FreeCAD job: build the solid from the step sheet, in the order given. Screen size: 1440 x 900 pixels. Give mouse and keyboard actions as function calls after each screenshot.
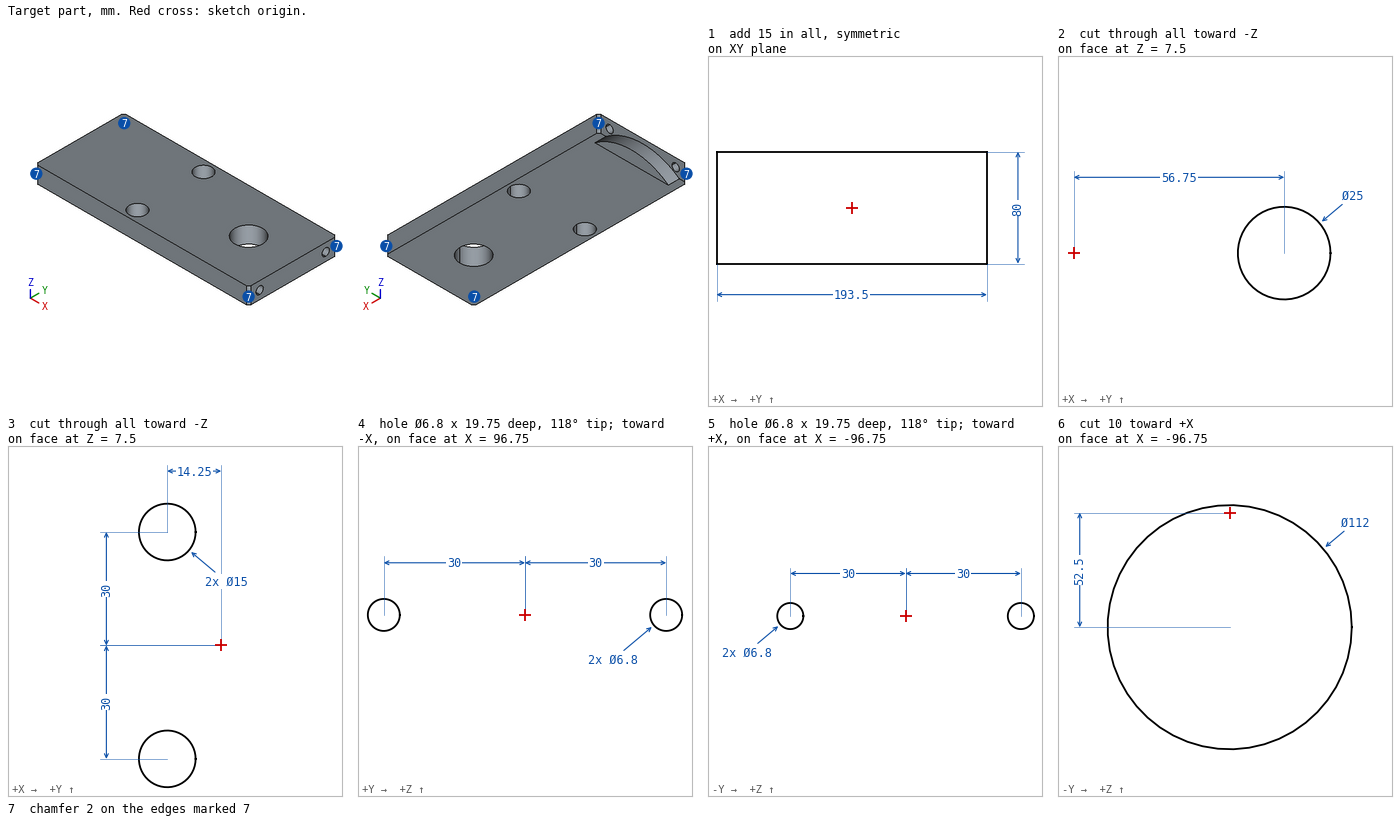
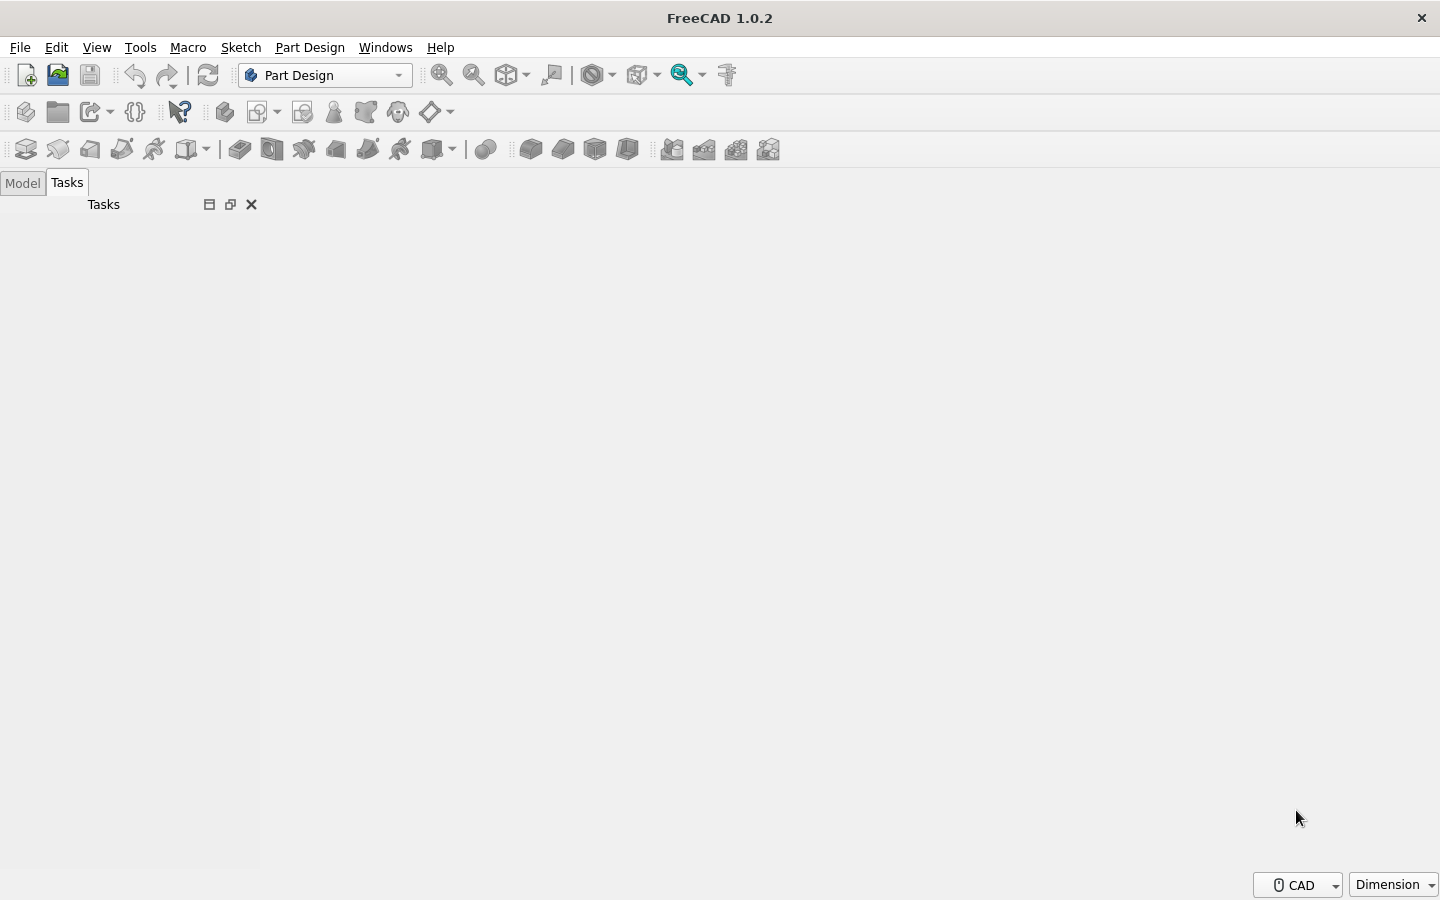
click(26, 76)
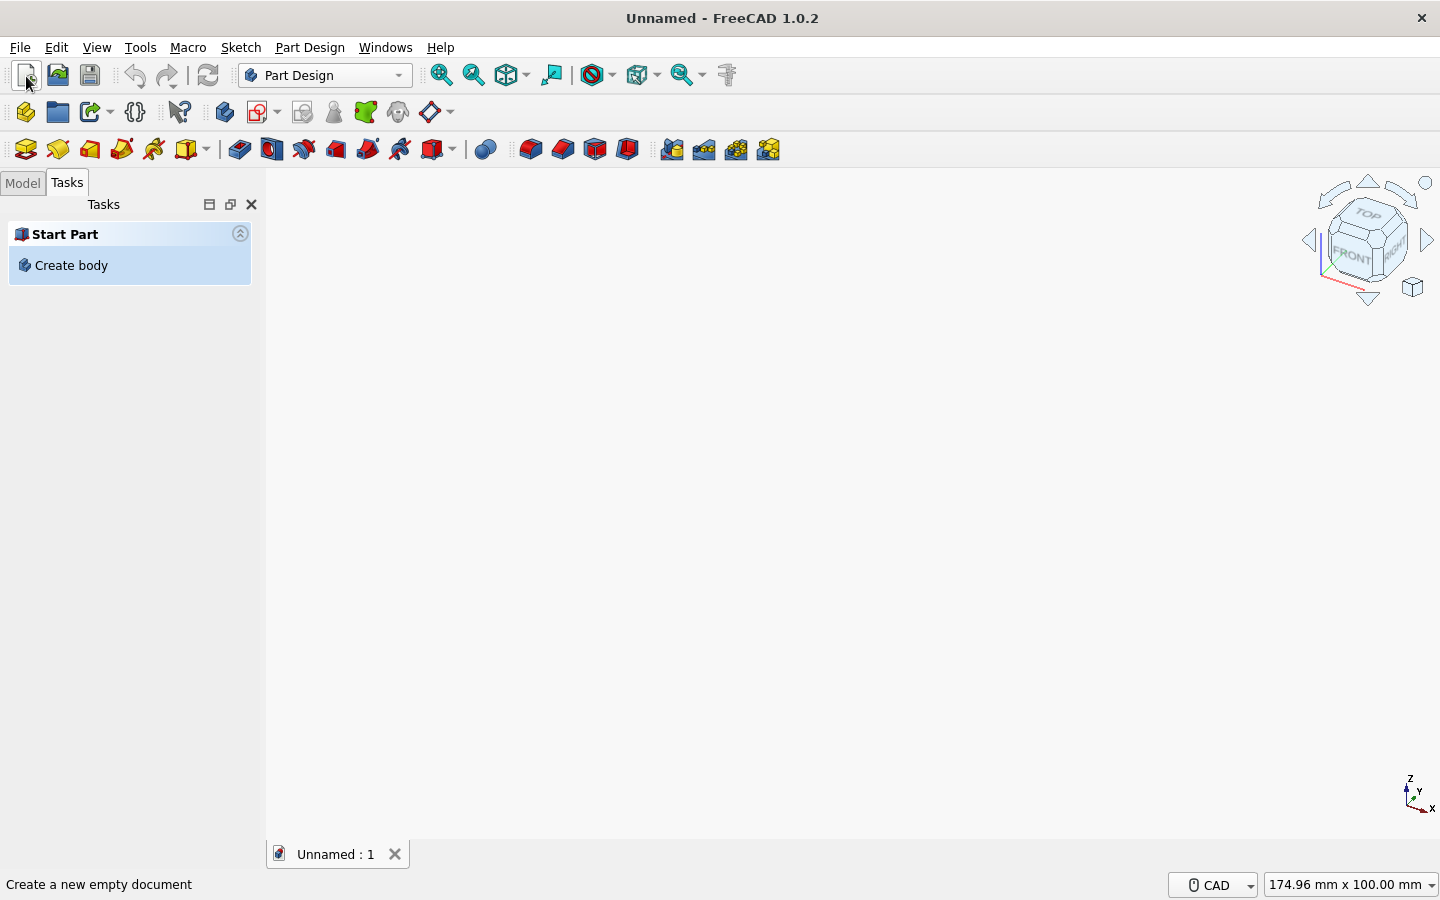
click(258, 112)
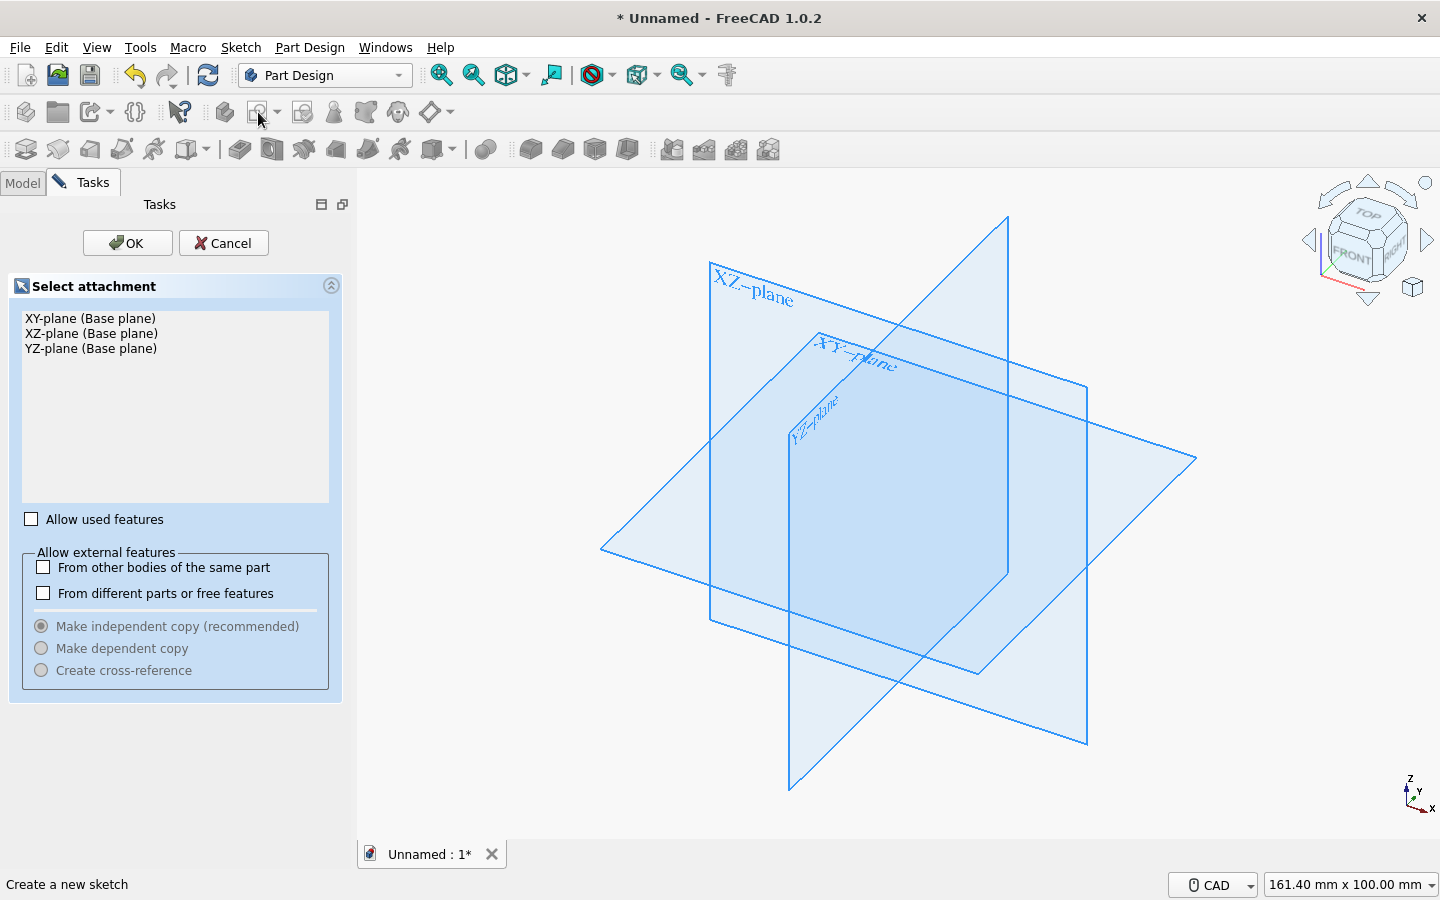
click(82, 318)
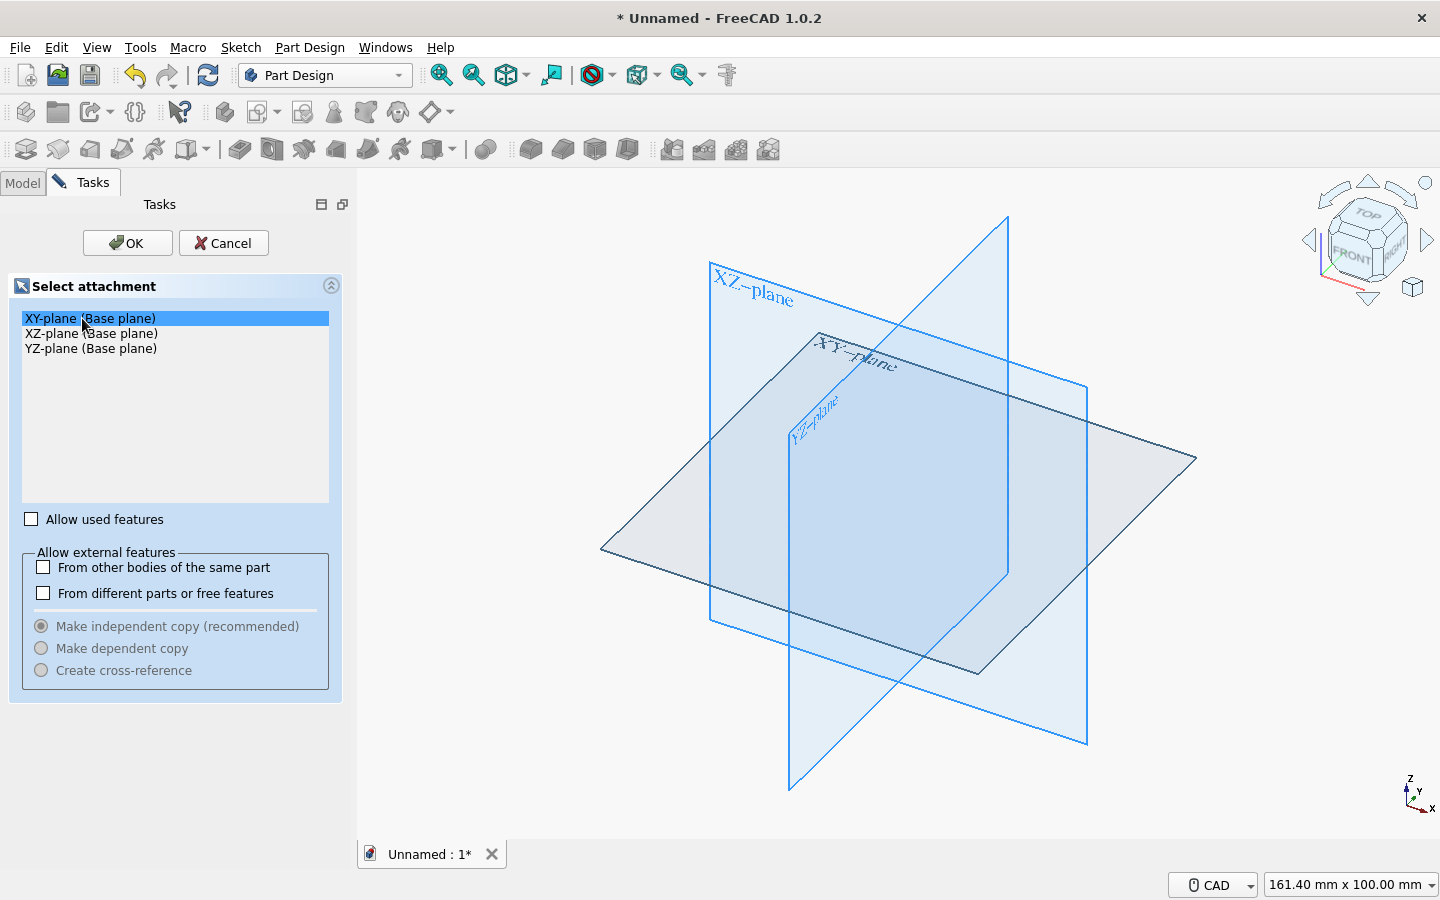
click(128, 243)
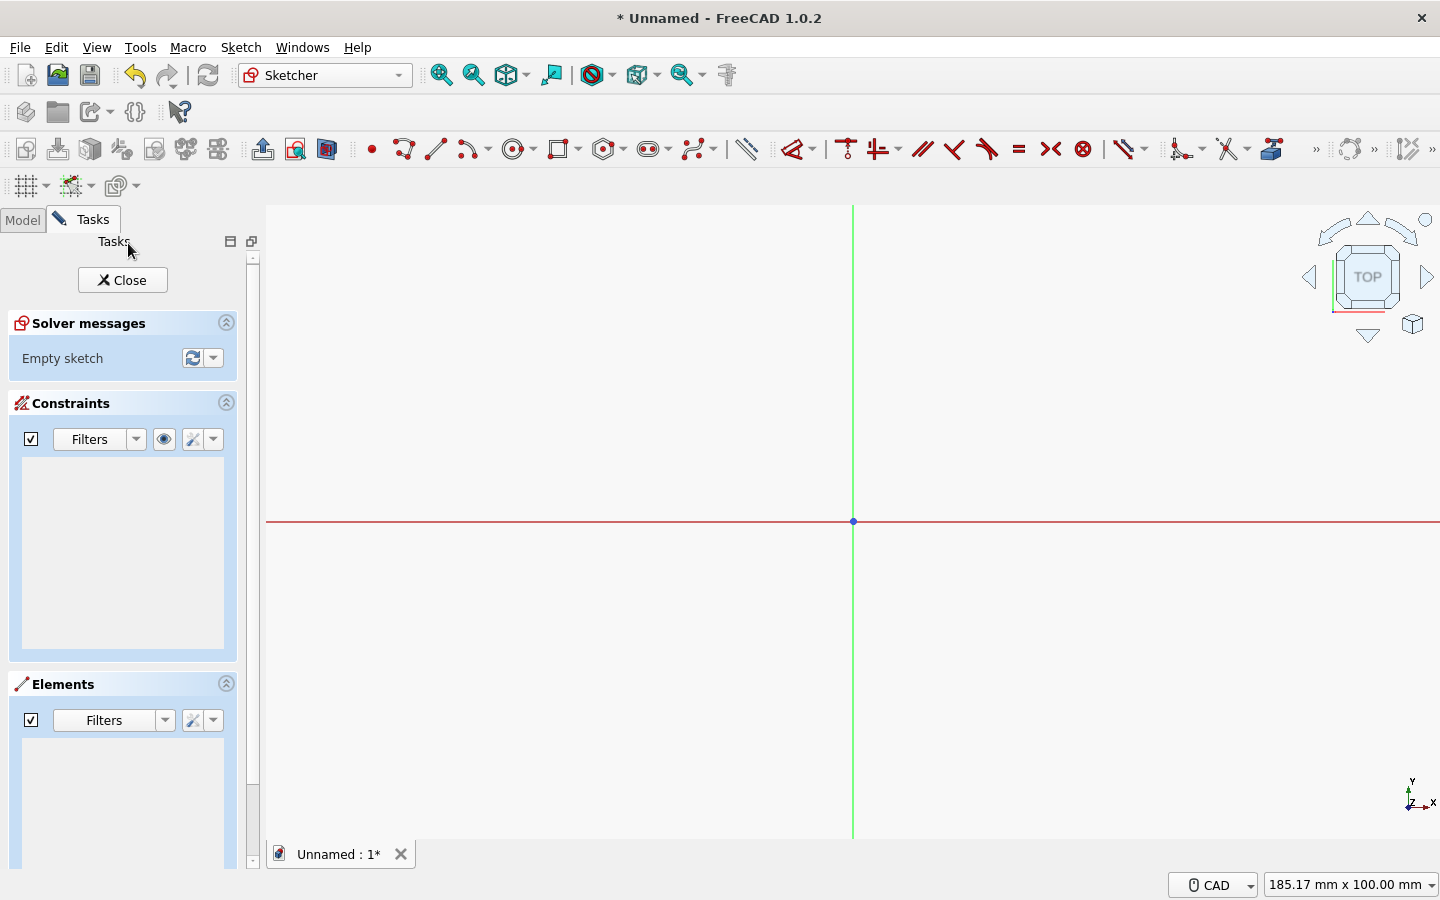
scroll(701, 522, down, 3)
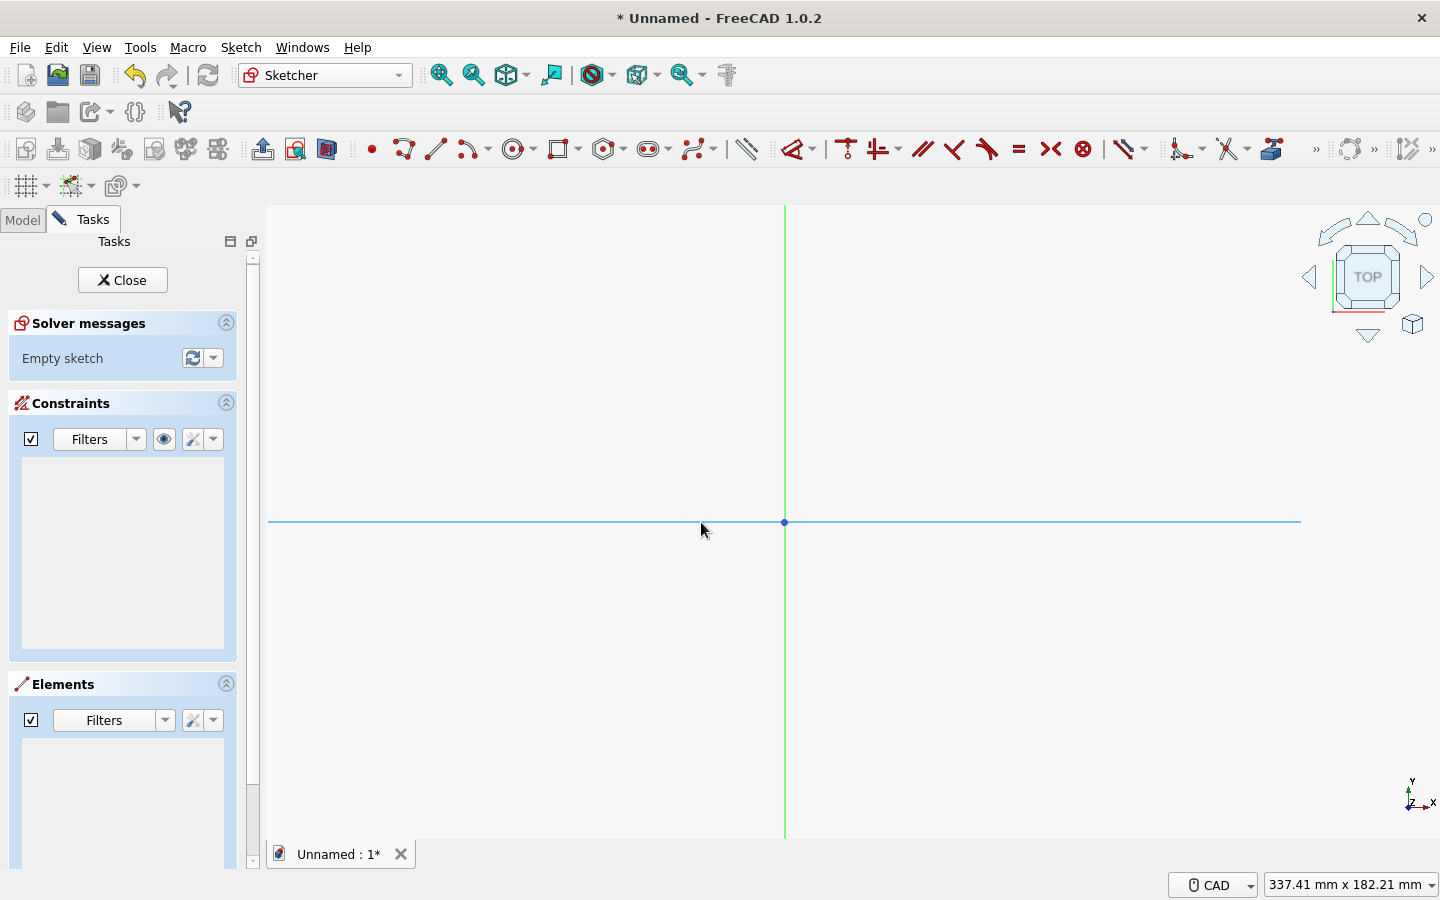
click(580, 150)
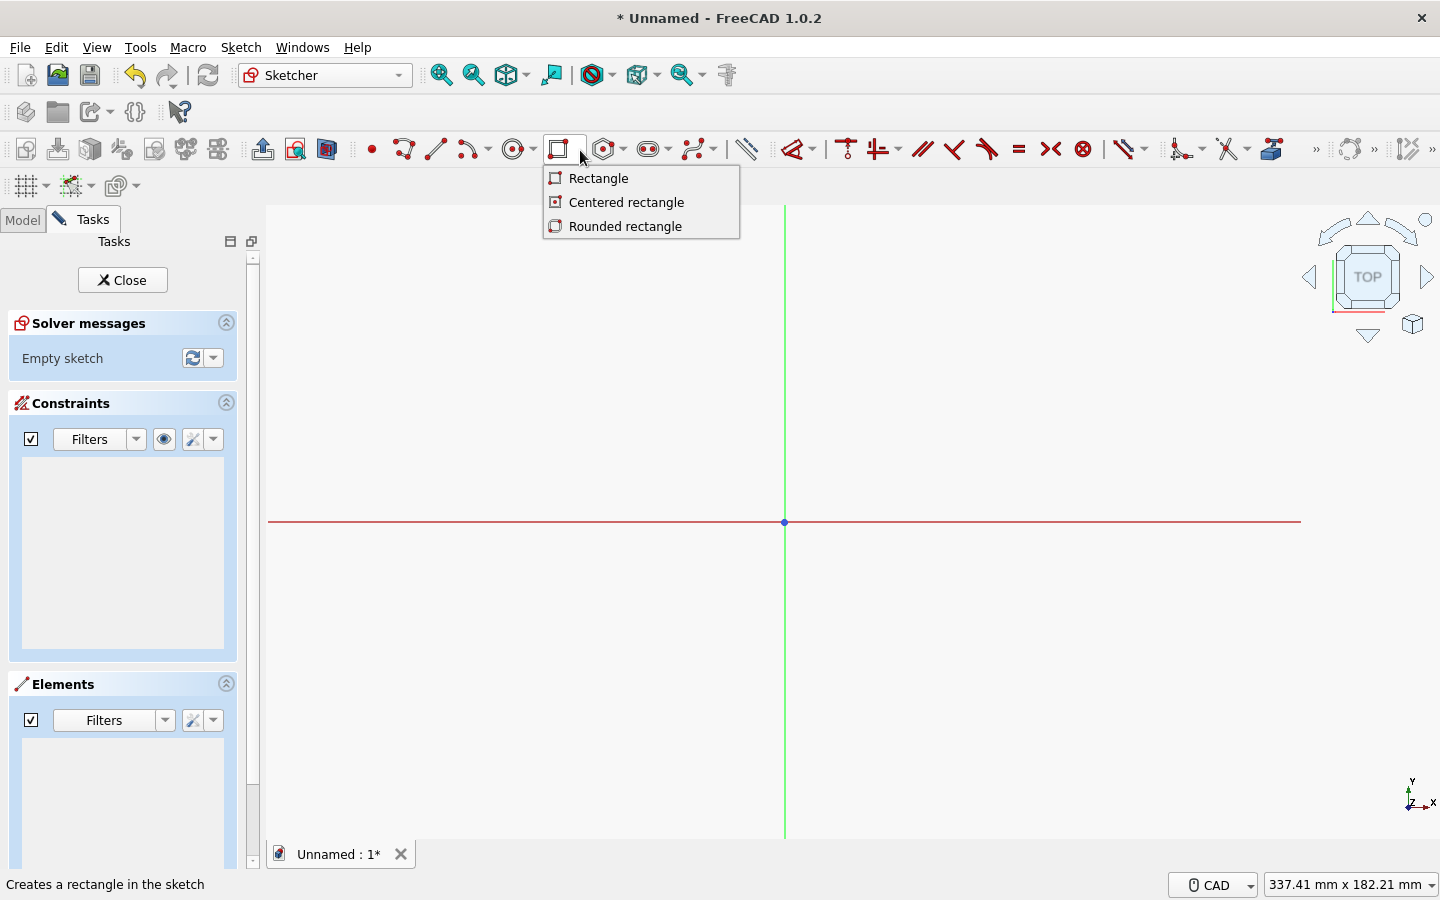
click(642, 202)